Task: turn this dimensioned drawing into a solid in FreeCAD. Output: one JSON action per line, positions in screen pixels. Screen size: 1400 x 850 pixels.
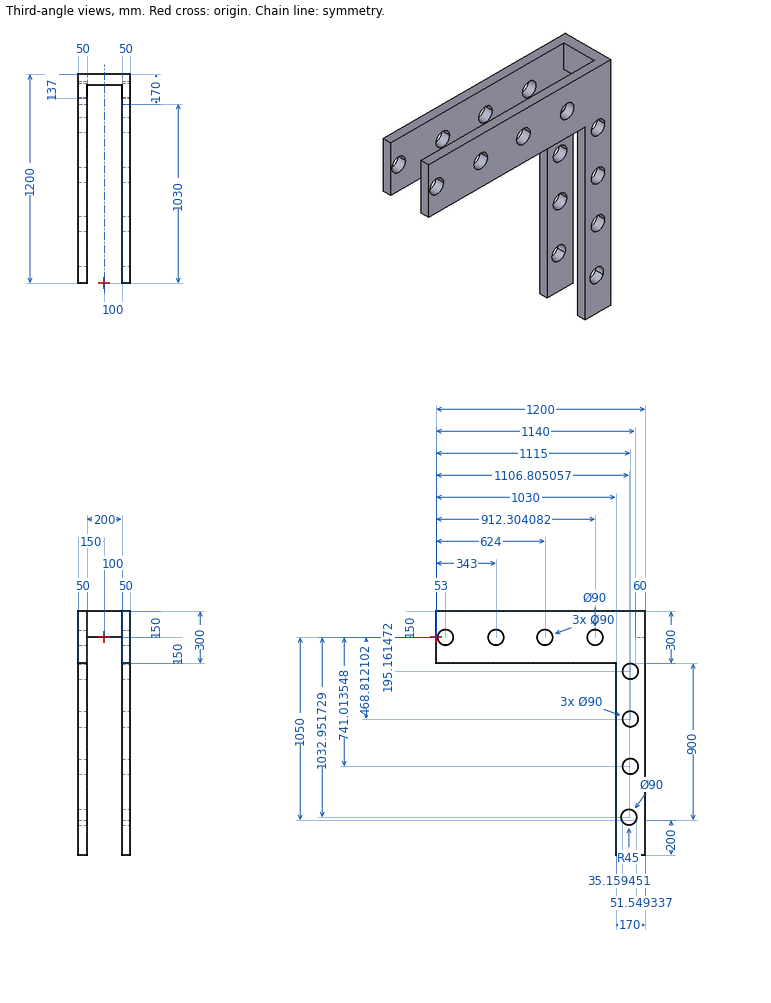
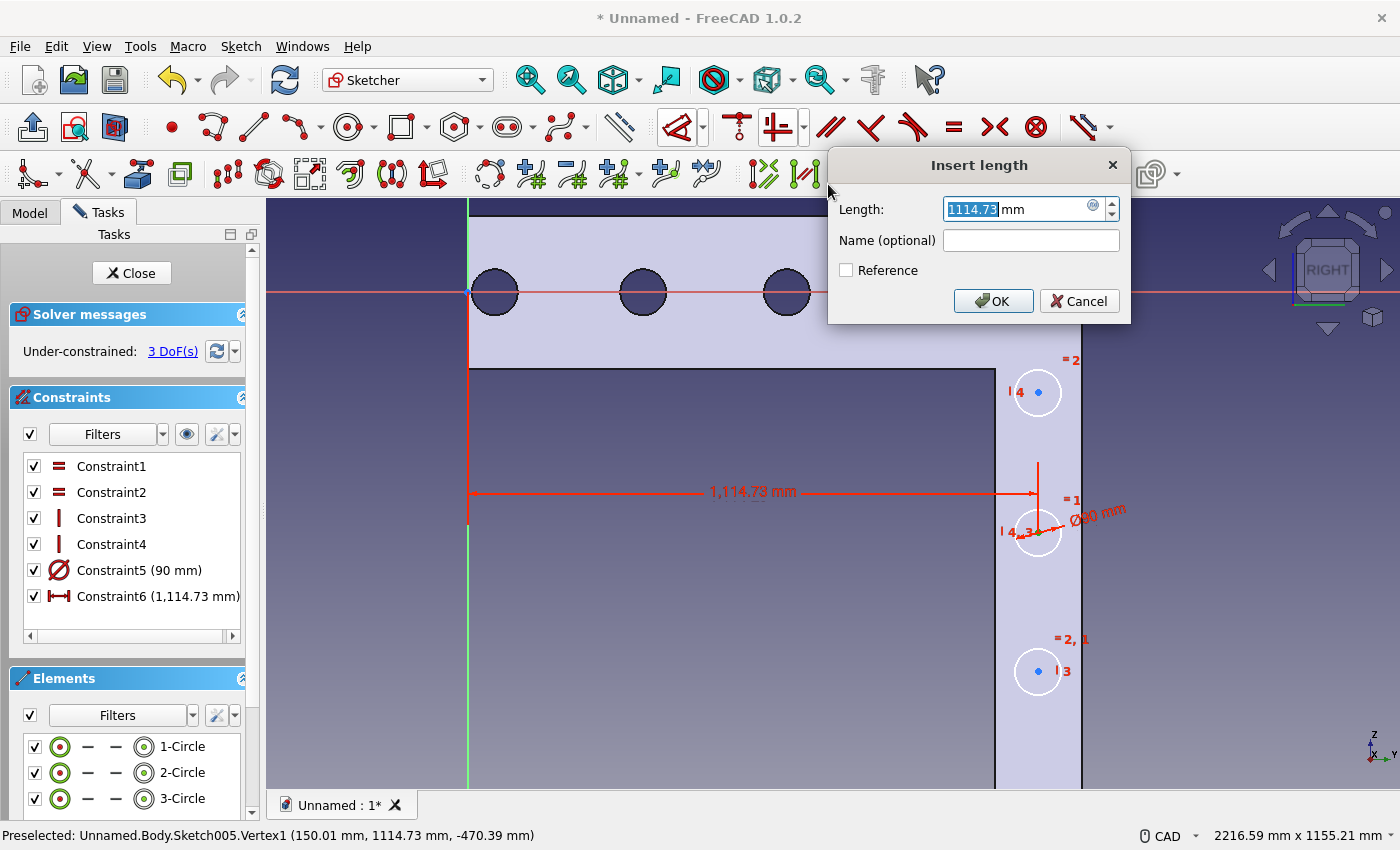
{"action": "type", "text": "1115"}
{"action": "key", "text": "Return"}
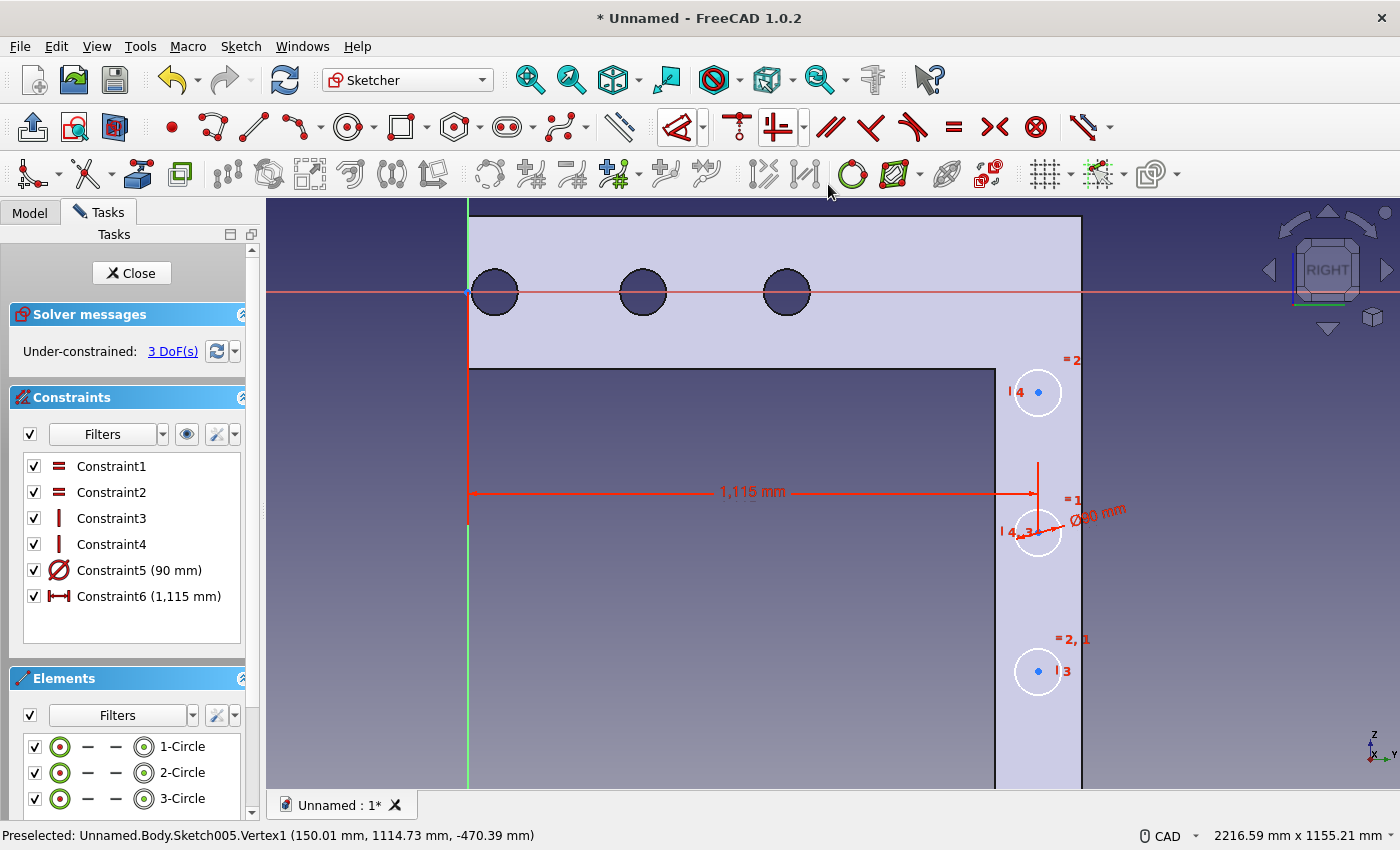
{"action": "left_click", "coordinate": [1038, 533]}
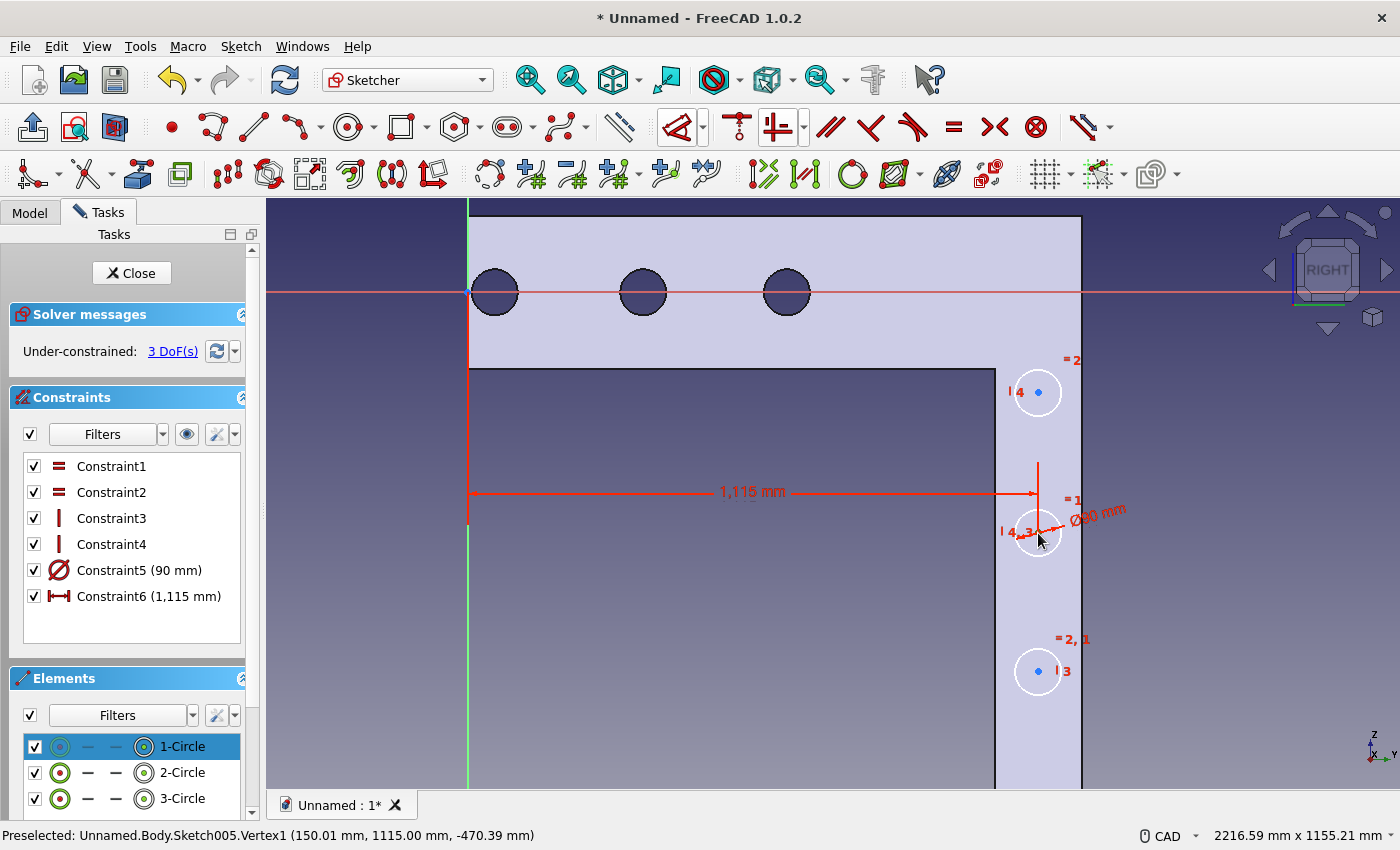
{"action": "key", "text": "i"}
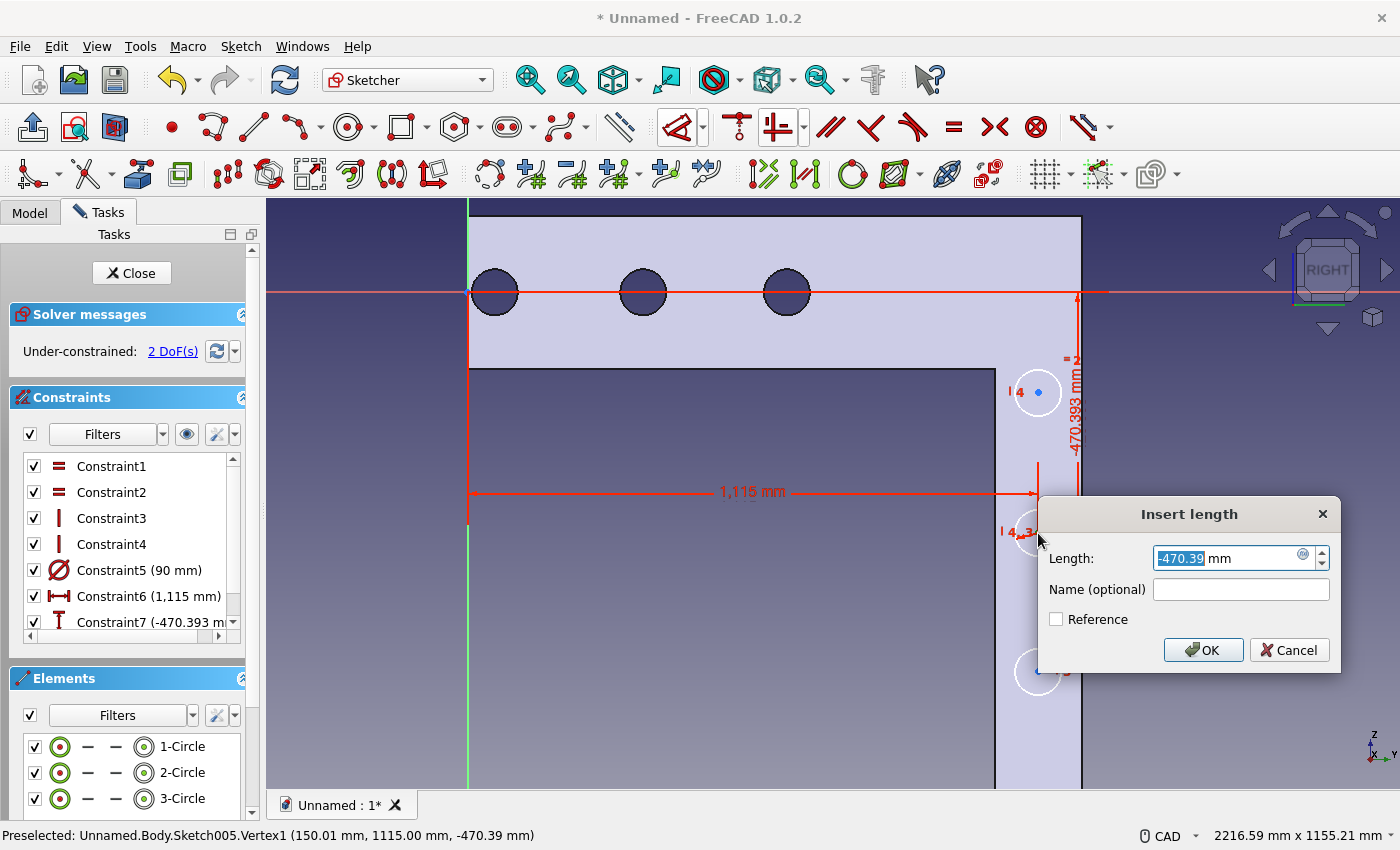
{"action": "type", "text": "-468.812102"}
{"action": "key", "text": "Return"}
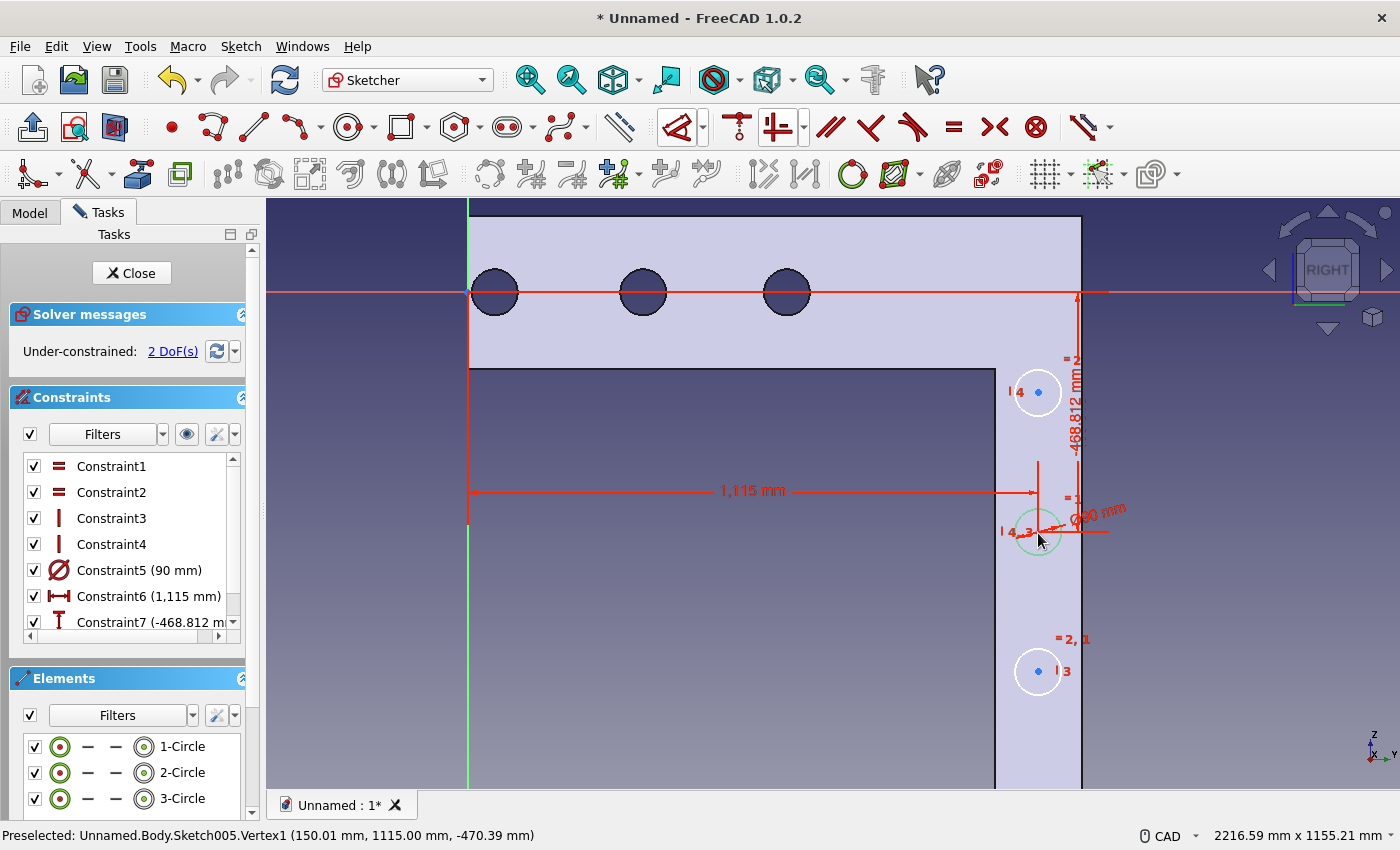
{"action": "left_click", "coordinate": [1038, 672]}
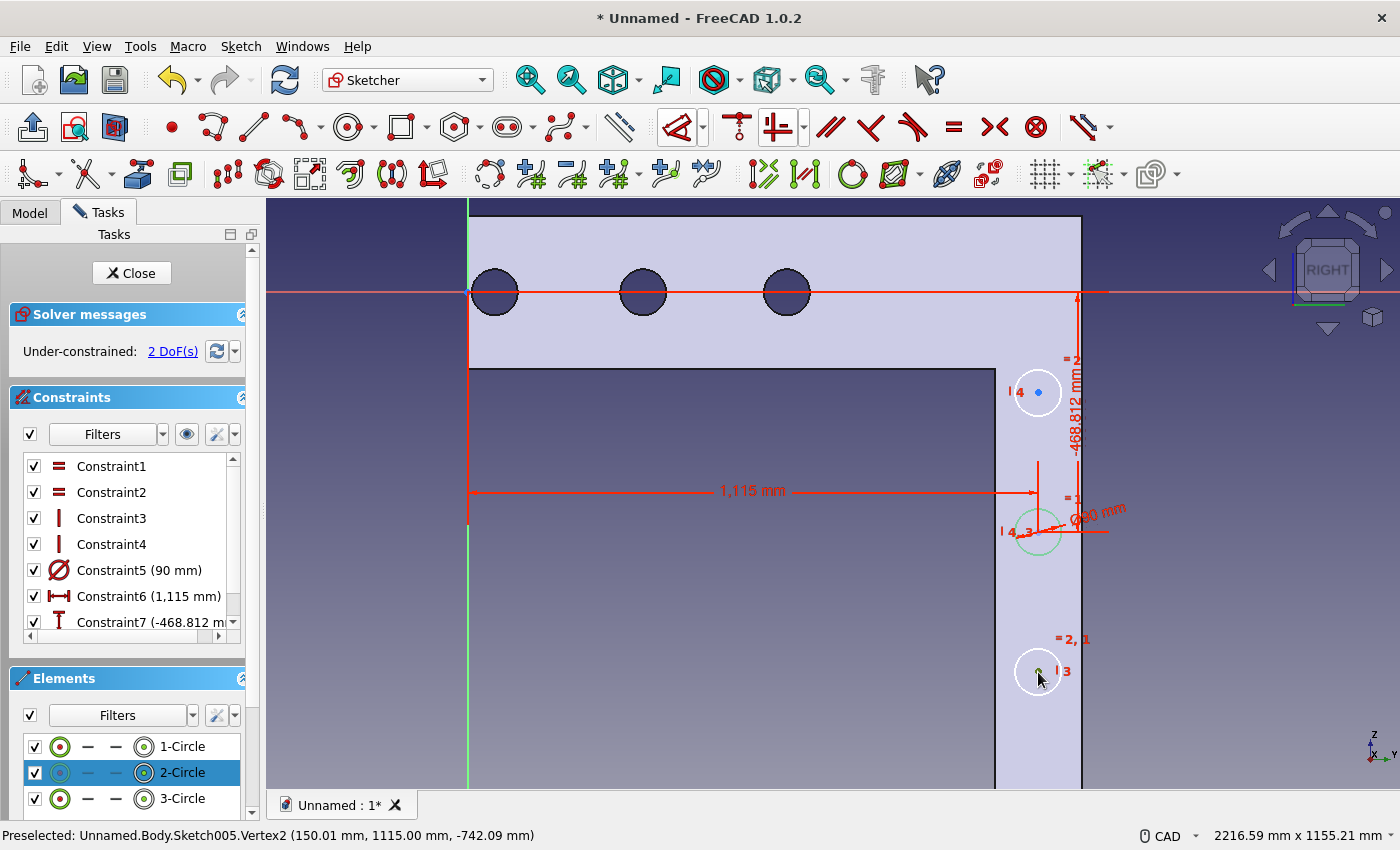
{"action": "key", "text": "i"}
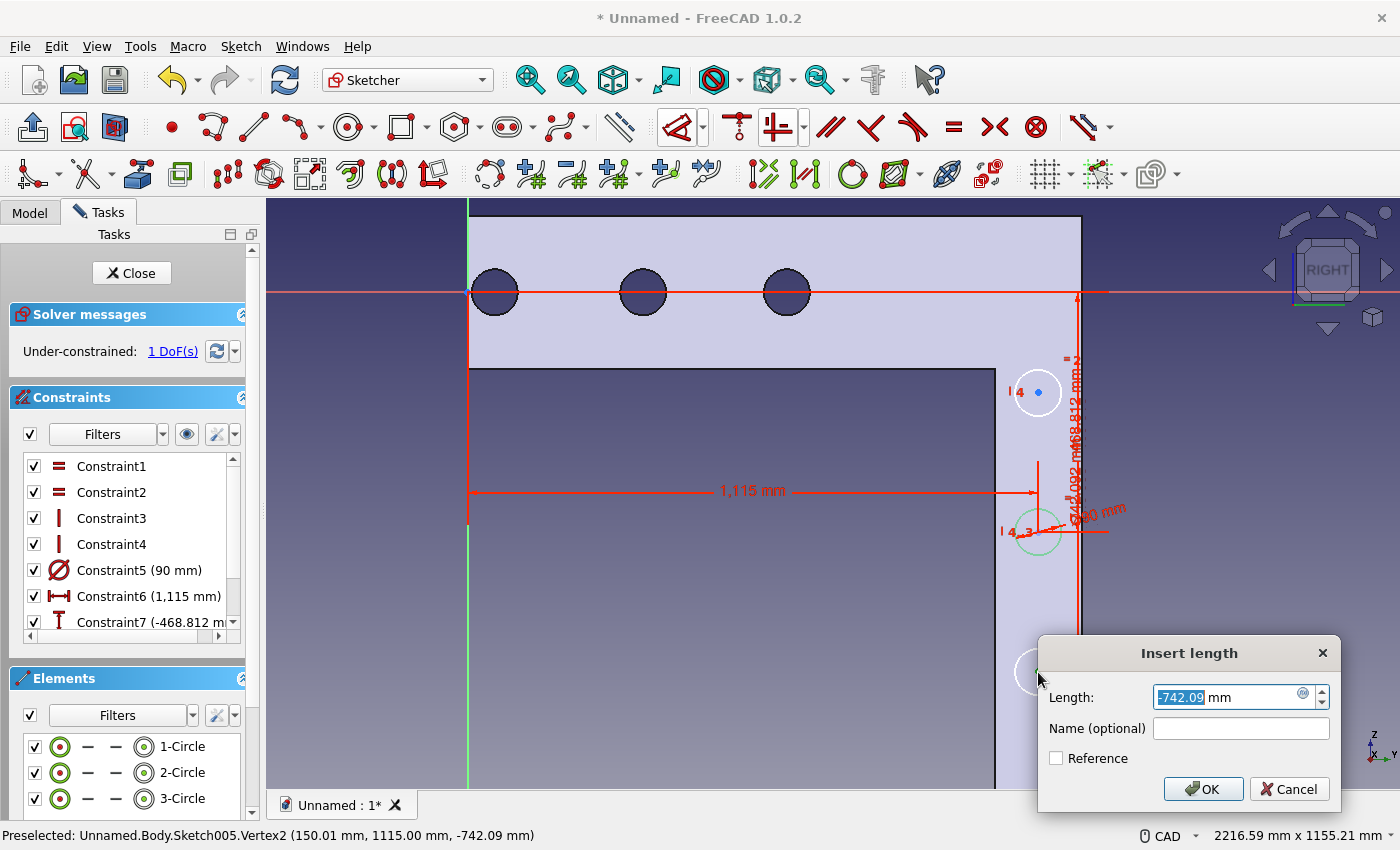
{"action": "type", "text": "-741.013548"}
{"action": "key", "text": "Return"}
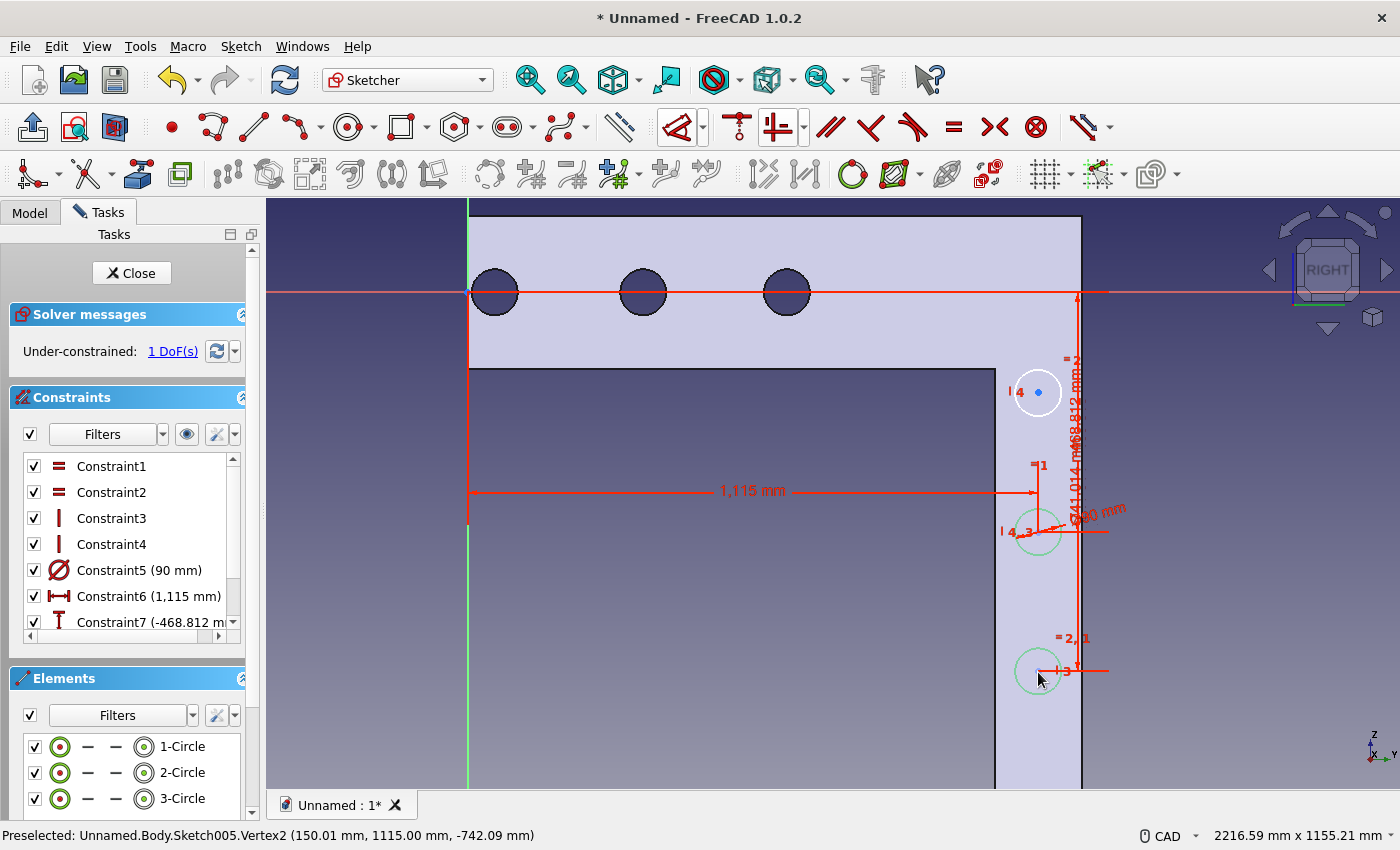
{"action": "left_click", "coordinate": [1038, 393]}